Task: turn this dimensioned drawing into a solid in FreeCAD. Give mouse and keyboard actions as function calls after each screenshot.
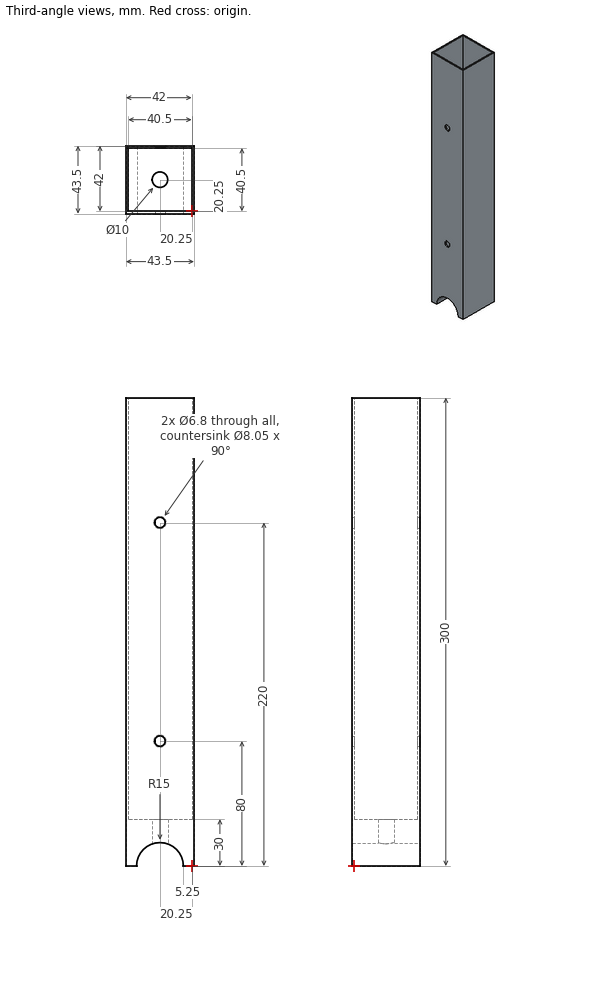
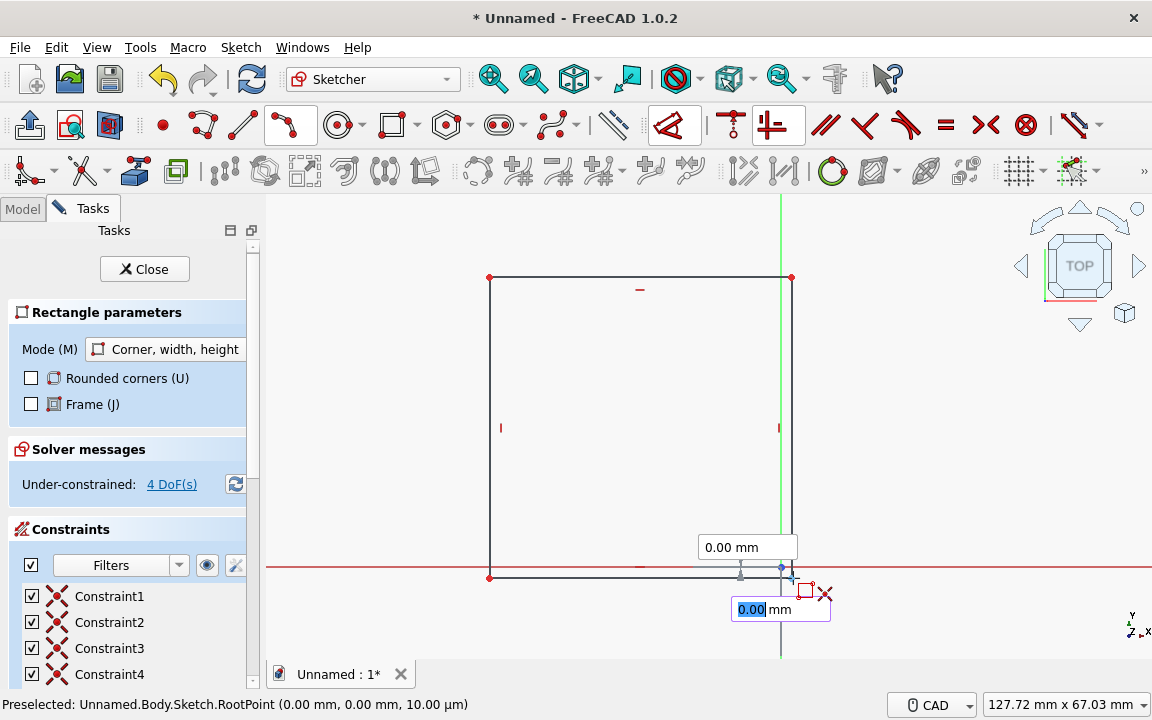
scroll(500, 286, up, 3)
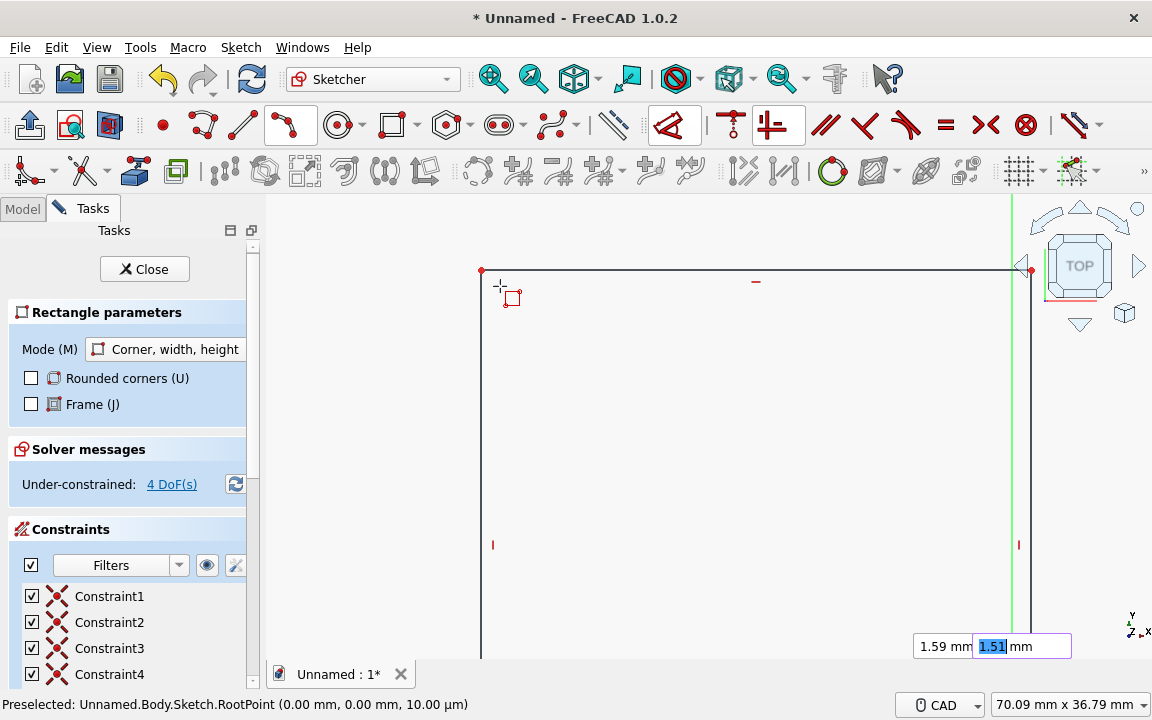
click(500, 286)
key(Escape)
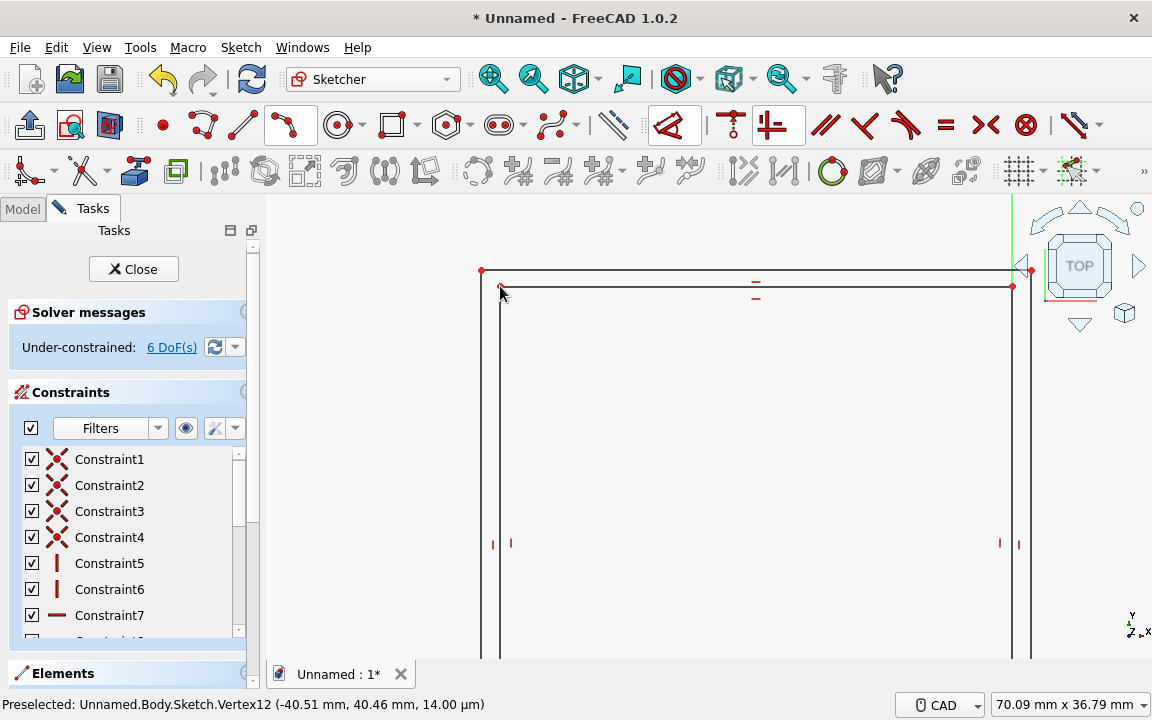
click(668, 126)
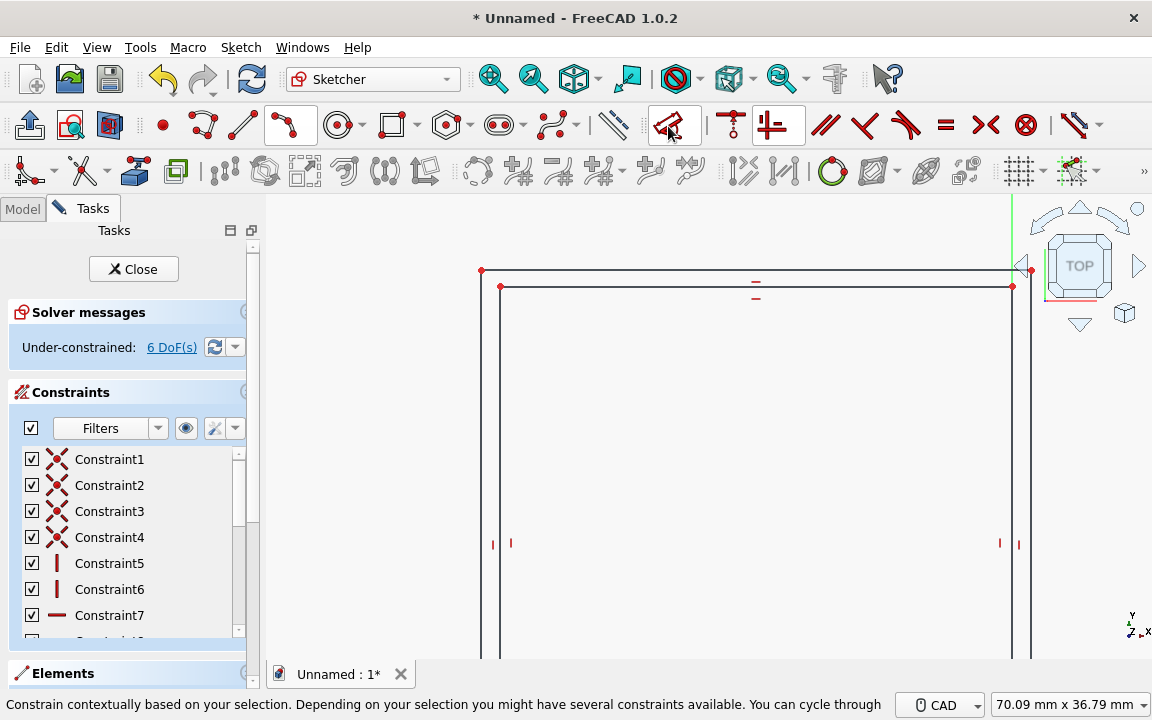
click(481, 270)
click(734, 236)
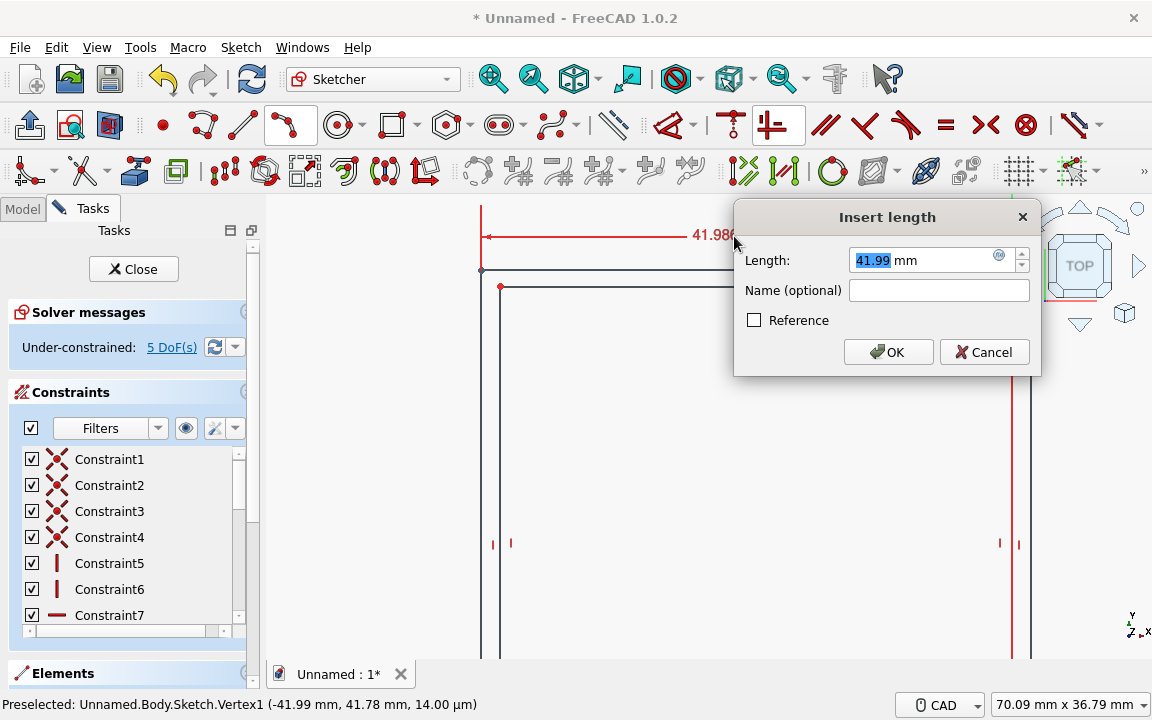
text(42)
key(Return)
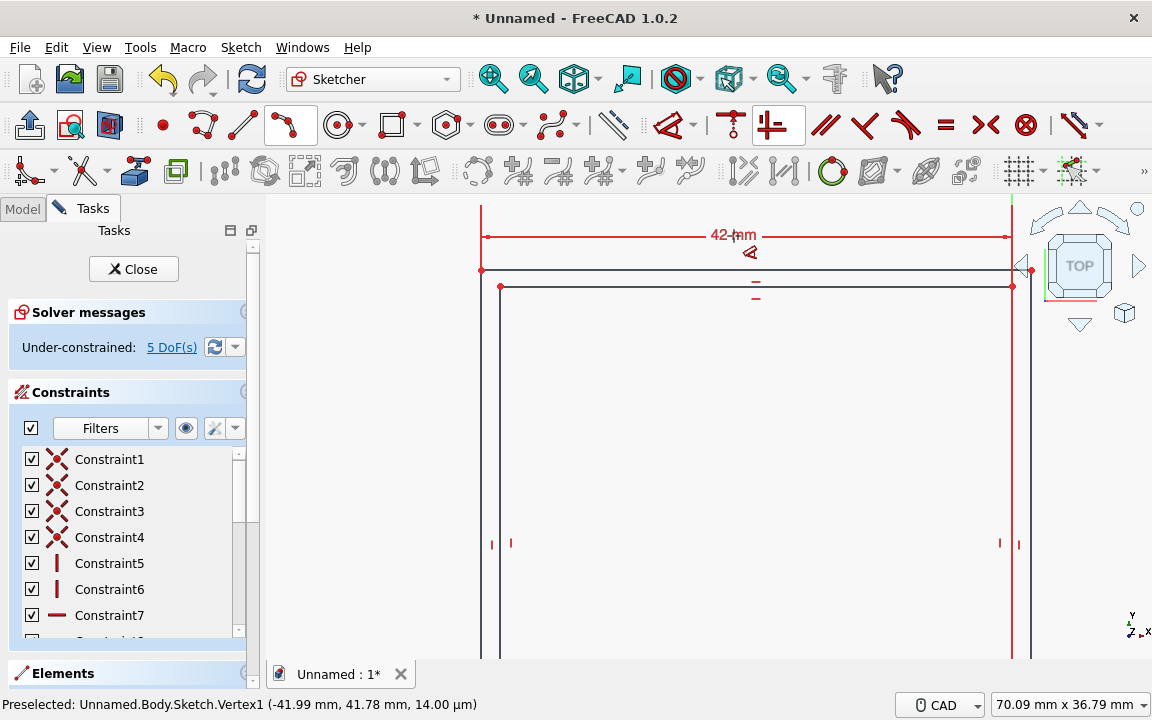
click(481, 270)
click(447, 451)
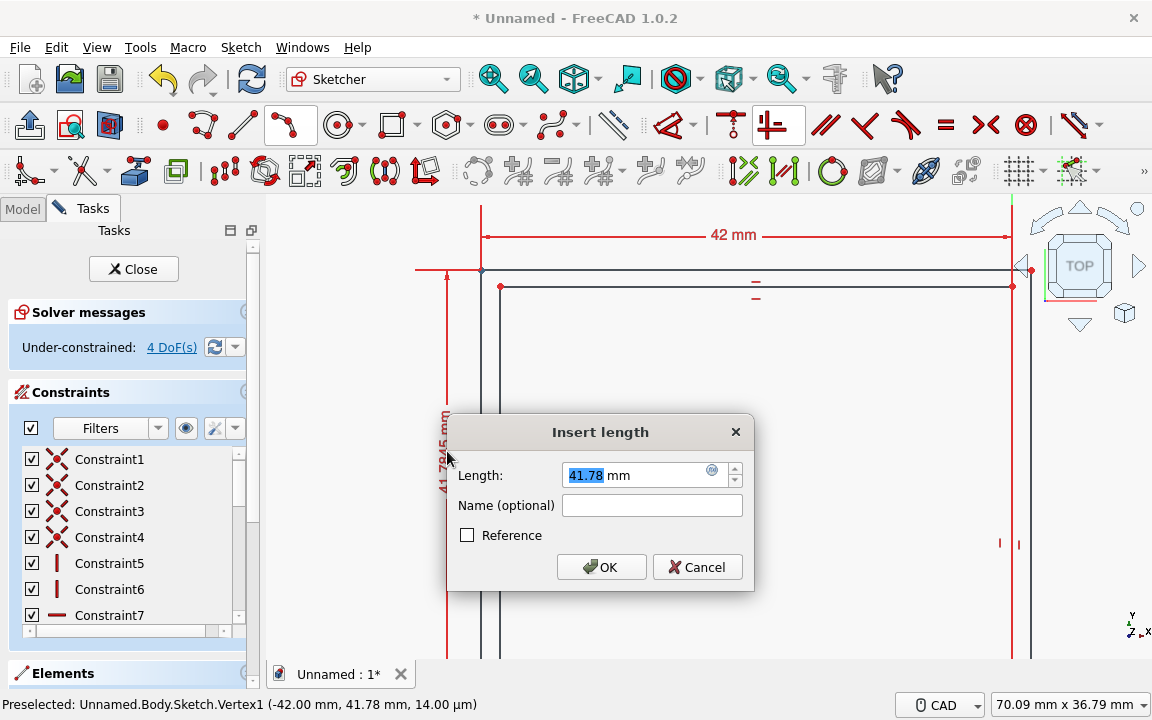
text(42)
key(Return)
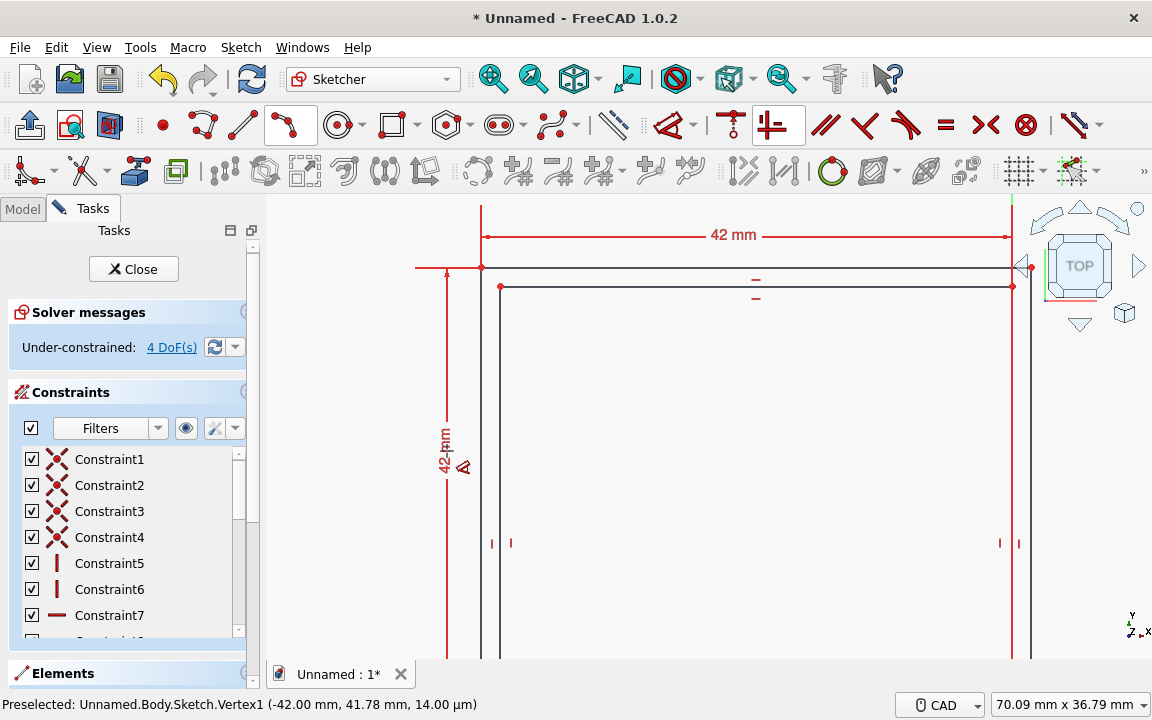
click(481, 433)
click(447, 366)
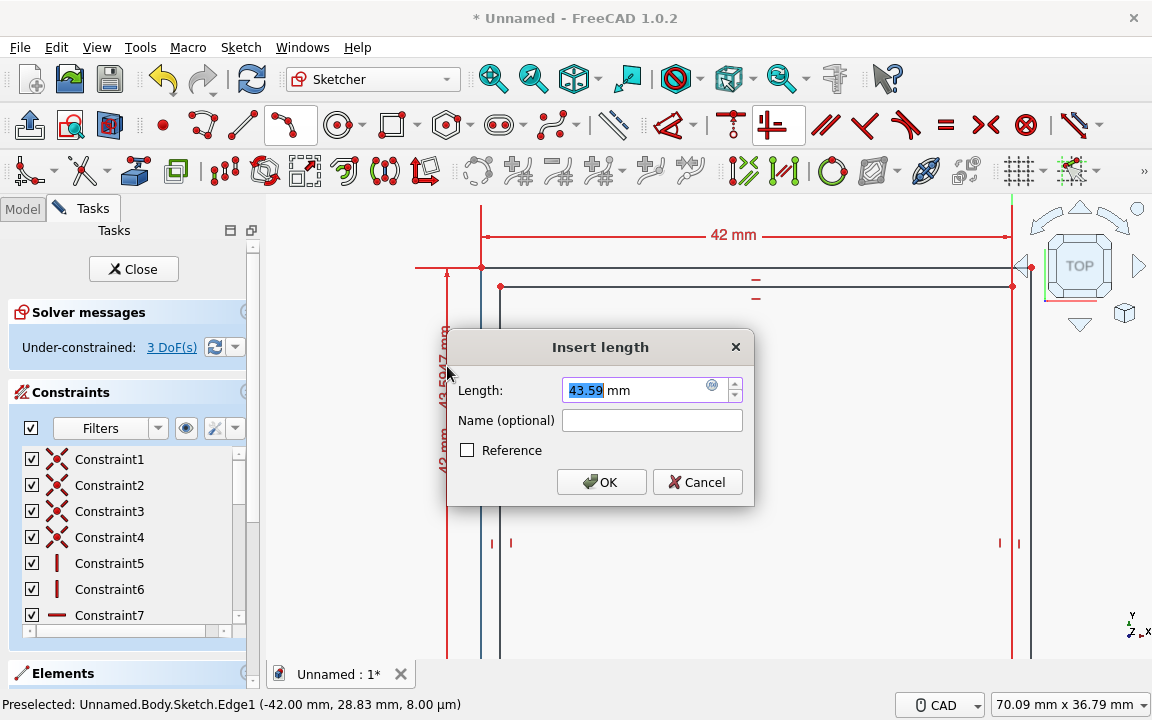
text(43.5)
key(Return)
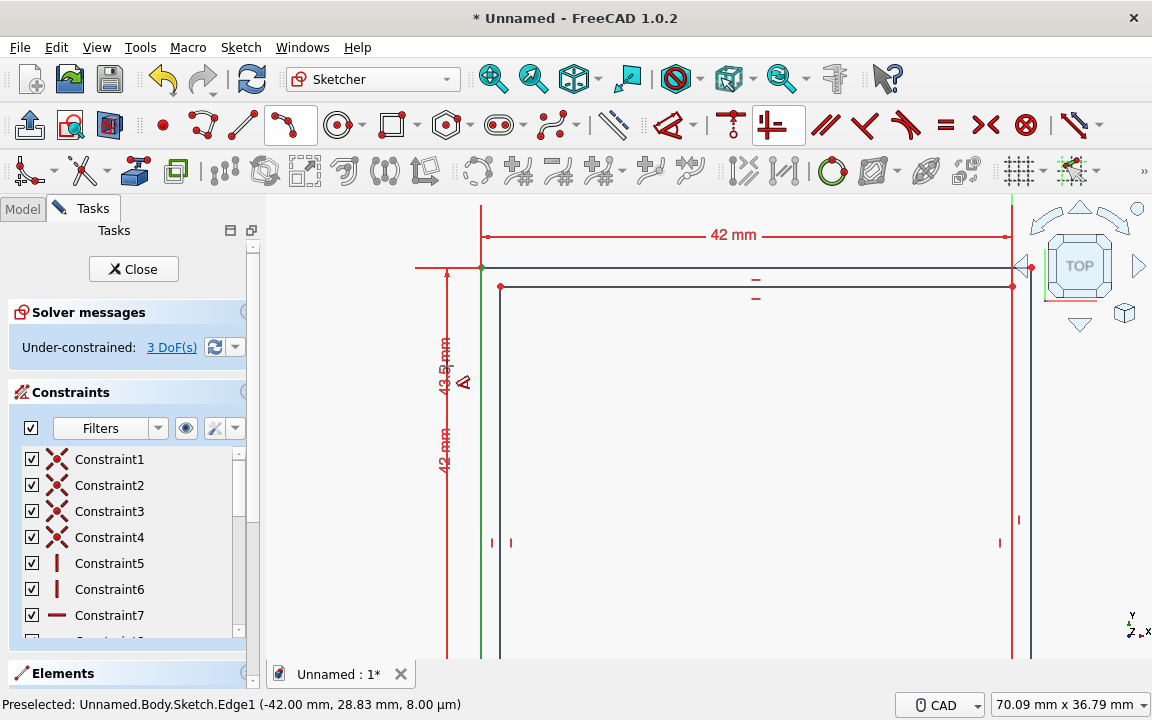
scroll(500, 285, down, 3)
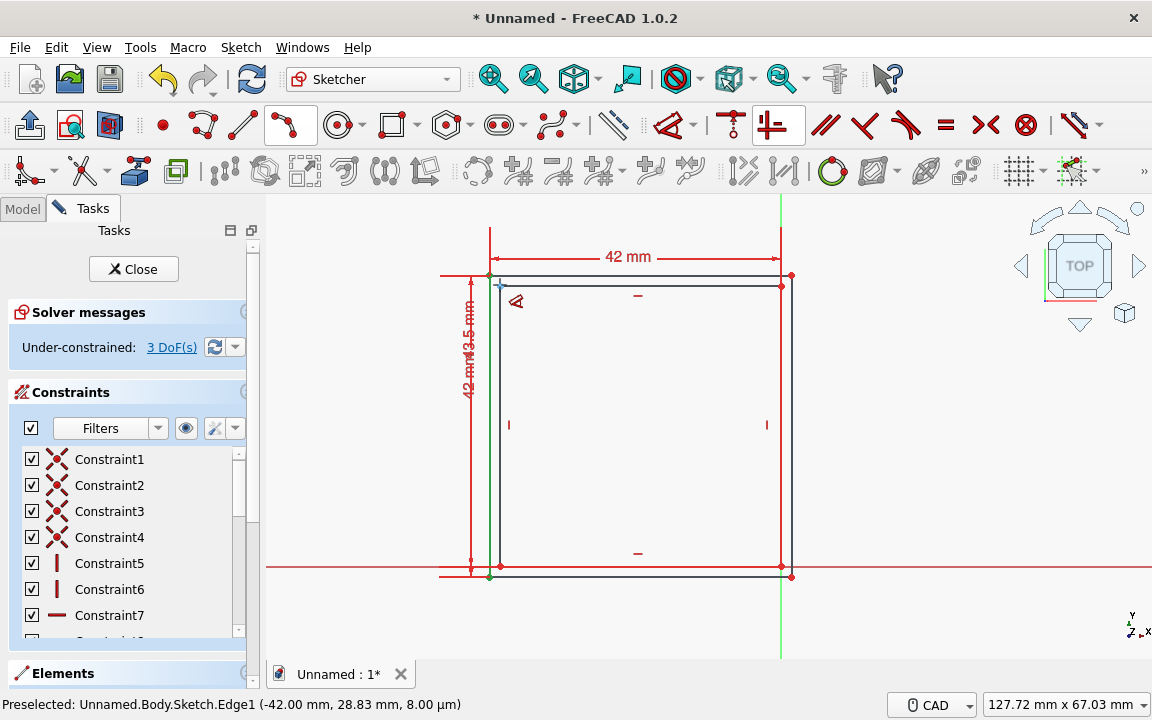
scroll(580, 577, up, 2)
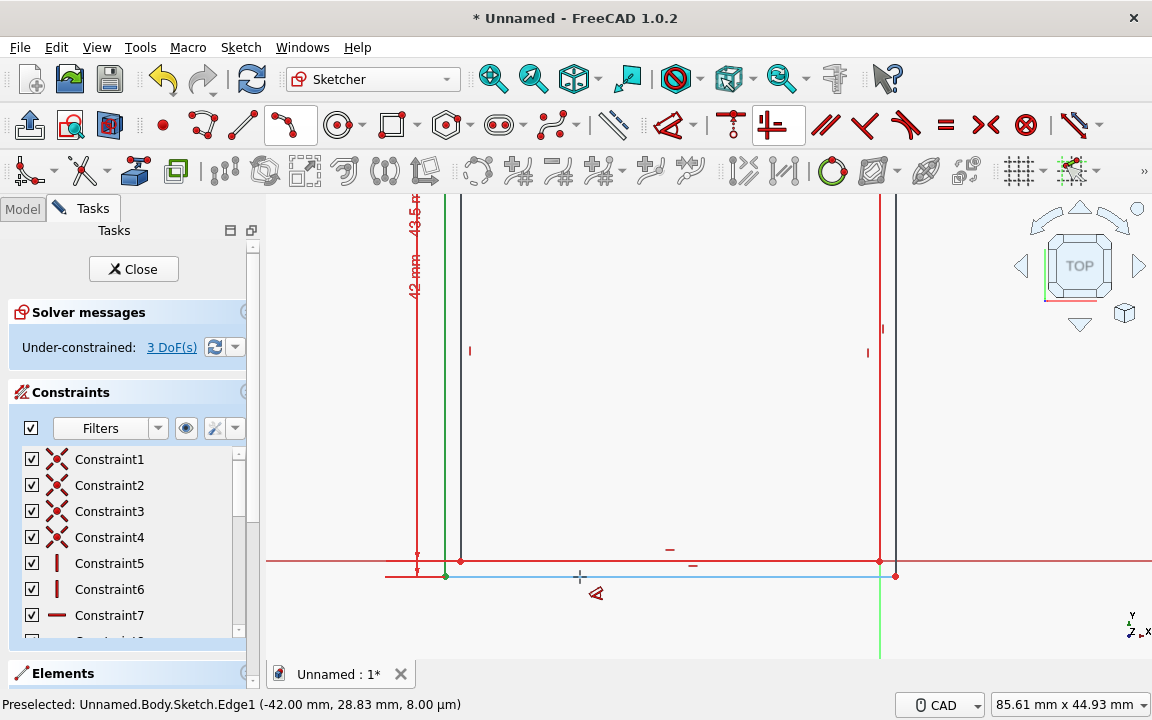
click(580, 577)
click(670, 611)